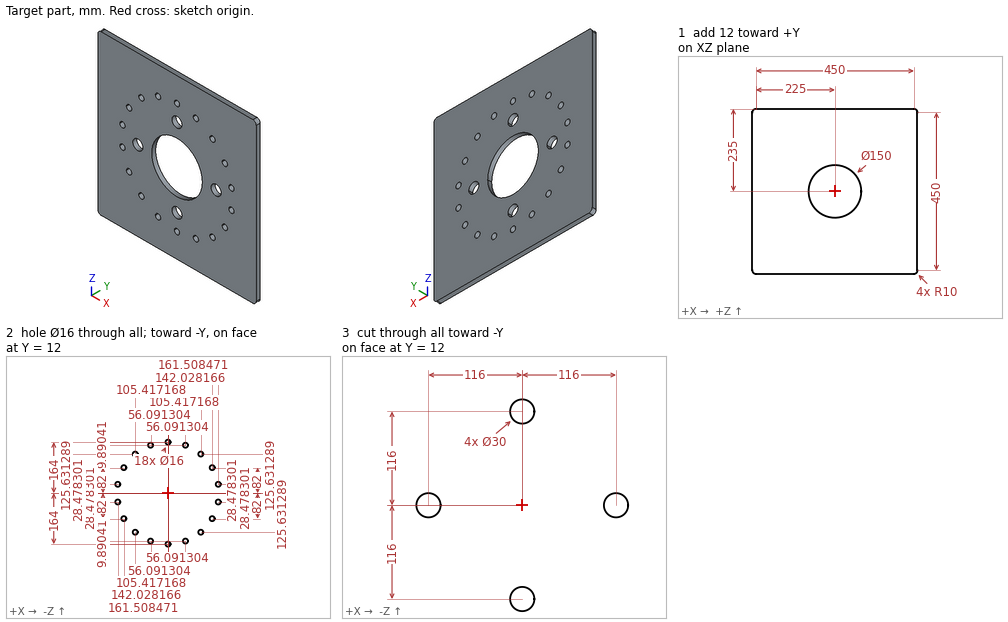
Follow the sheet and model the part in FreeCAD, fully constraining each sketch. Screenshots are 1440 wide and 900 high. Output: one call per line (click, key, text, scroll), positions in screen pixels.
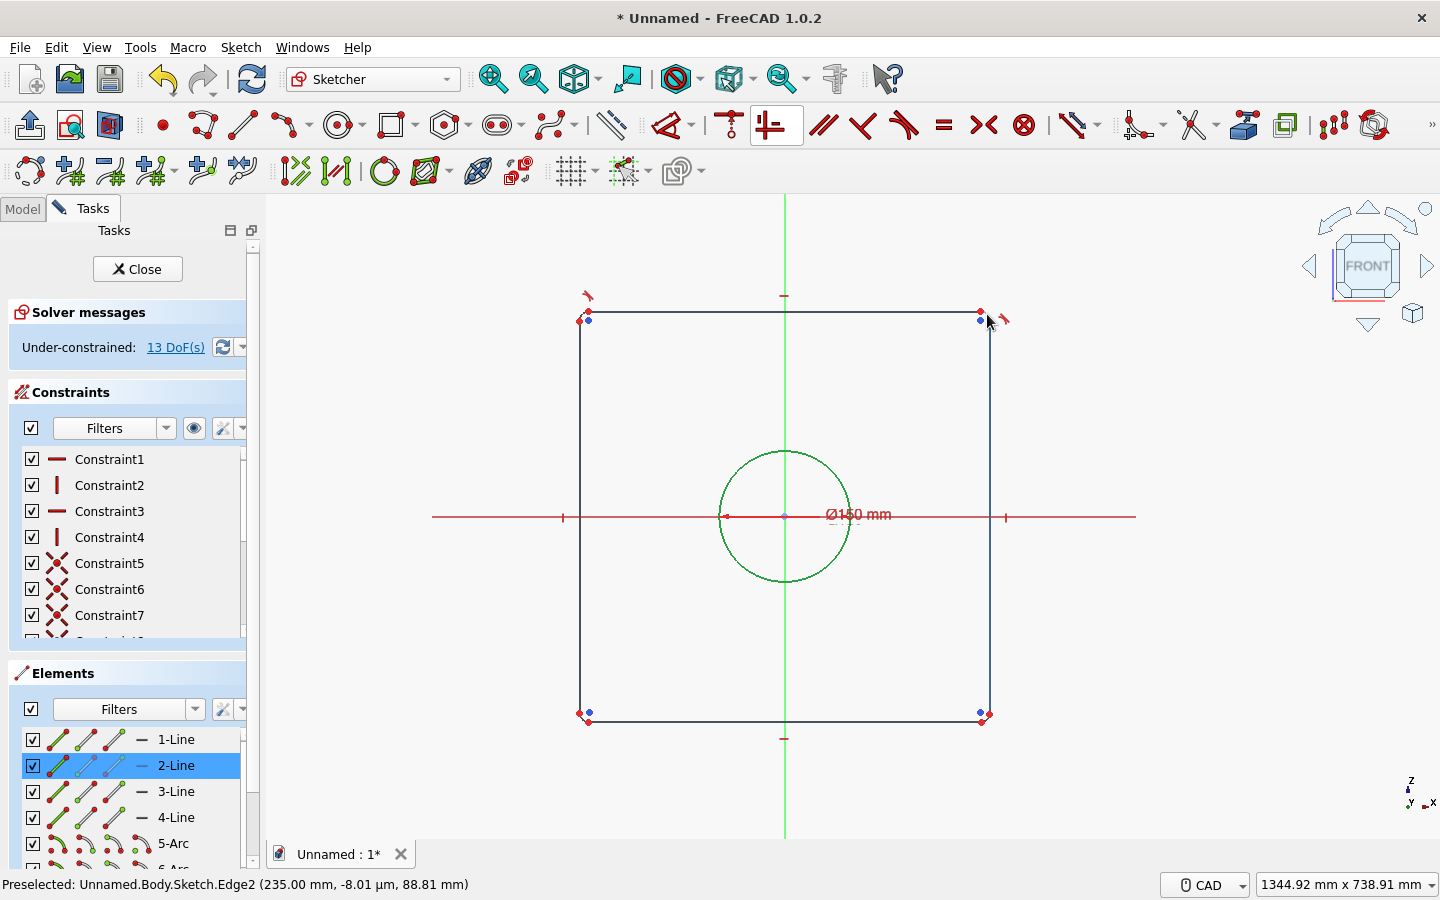
scroll(987, 720, up, 4)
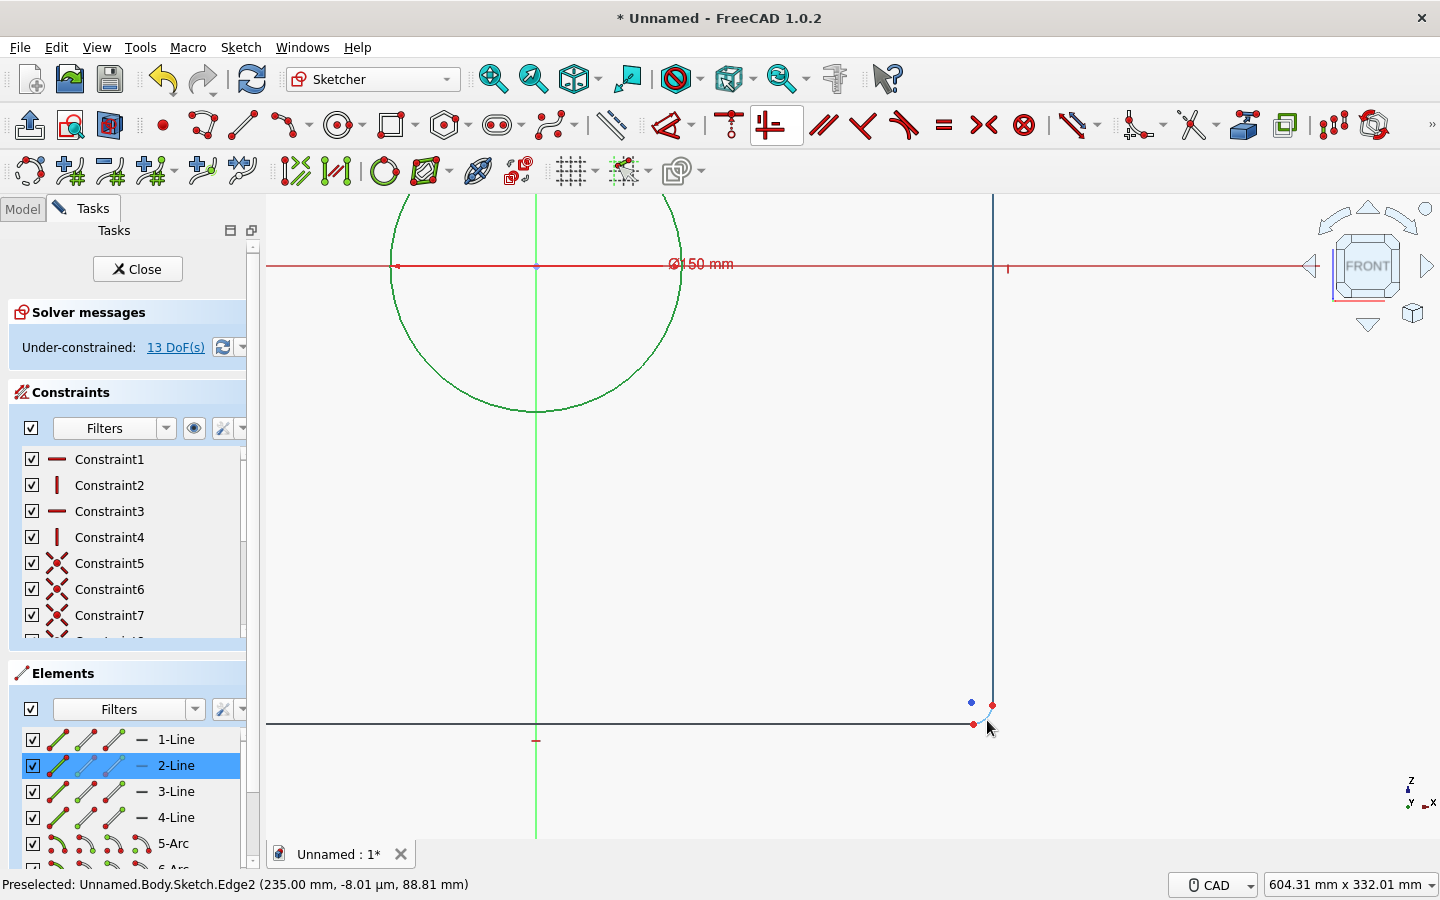
click(986, 718)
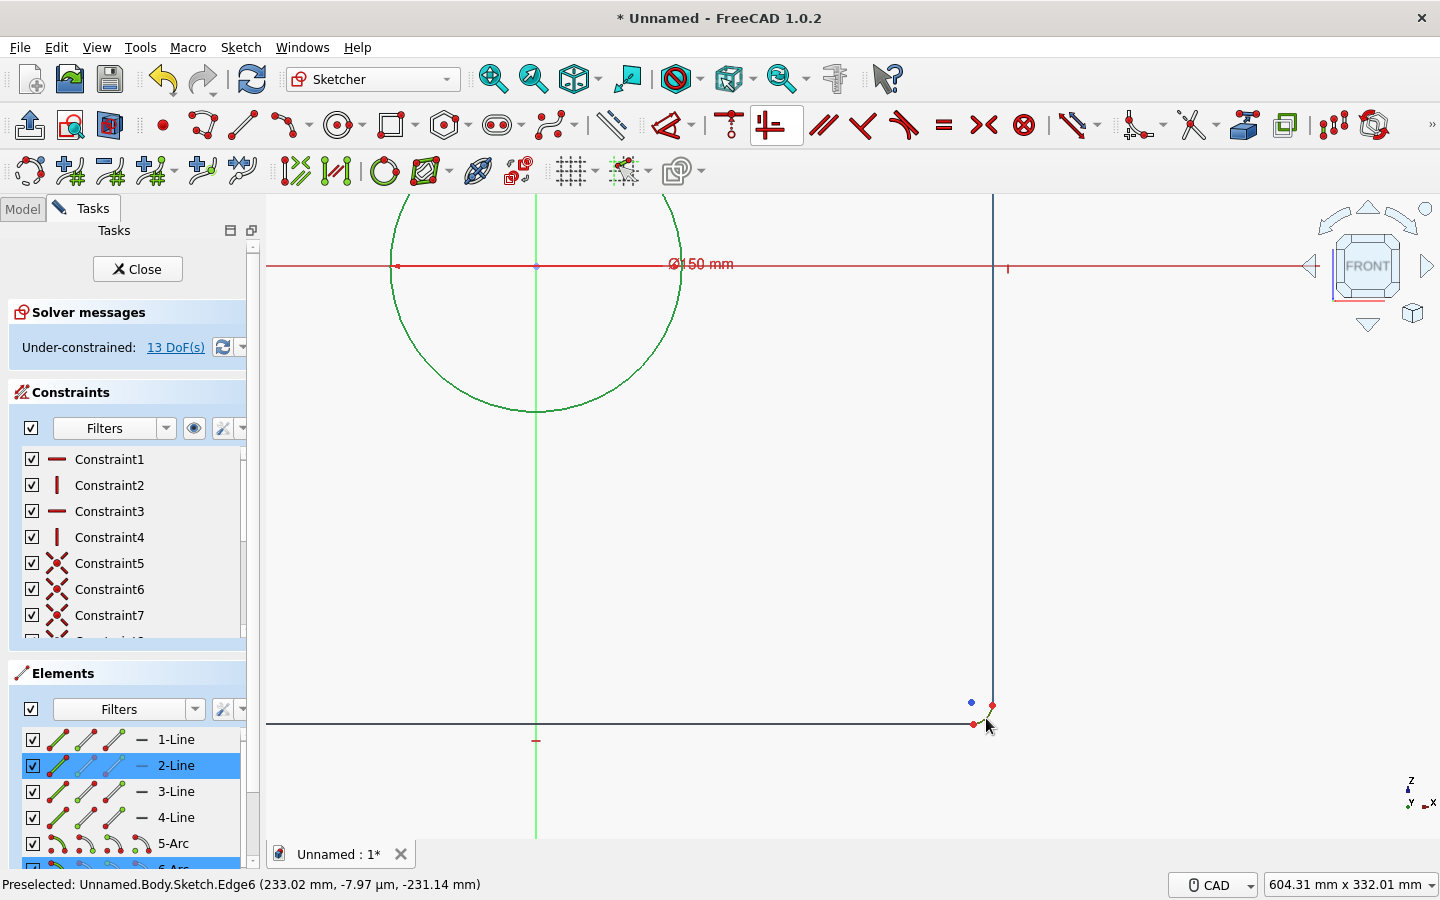
click(904, 126)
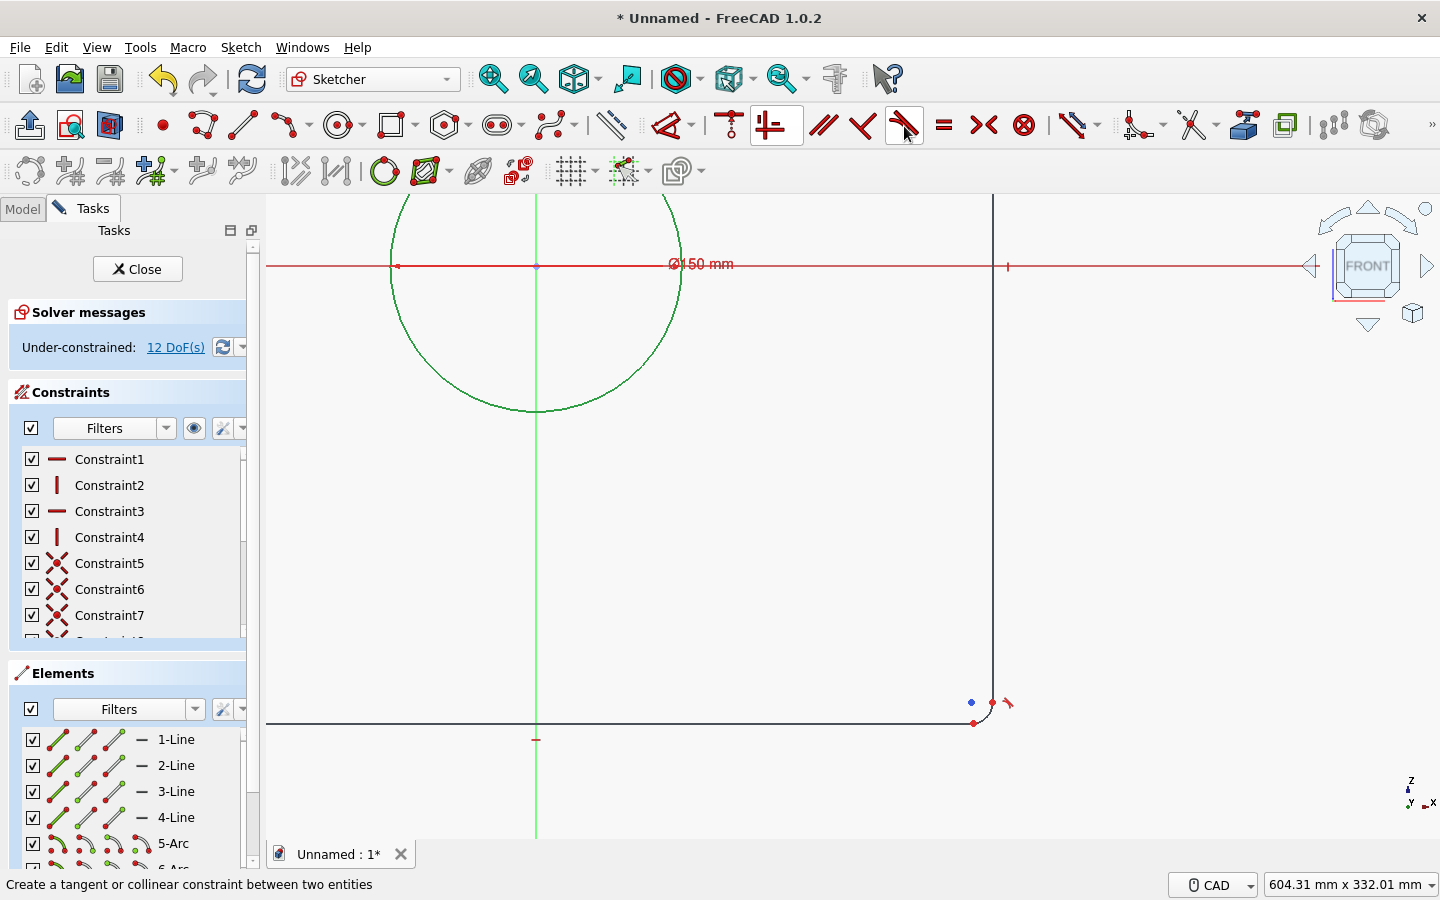
click(711, 724)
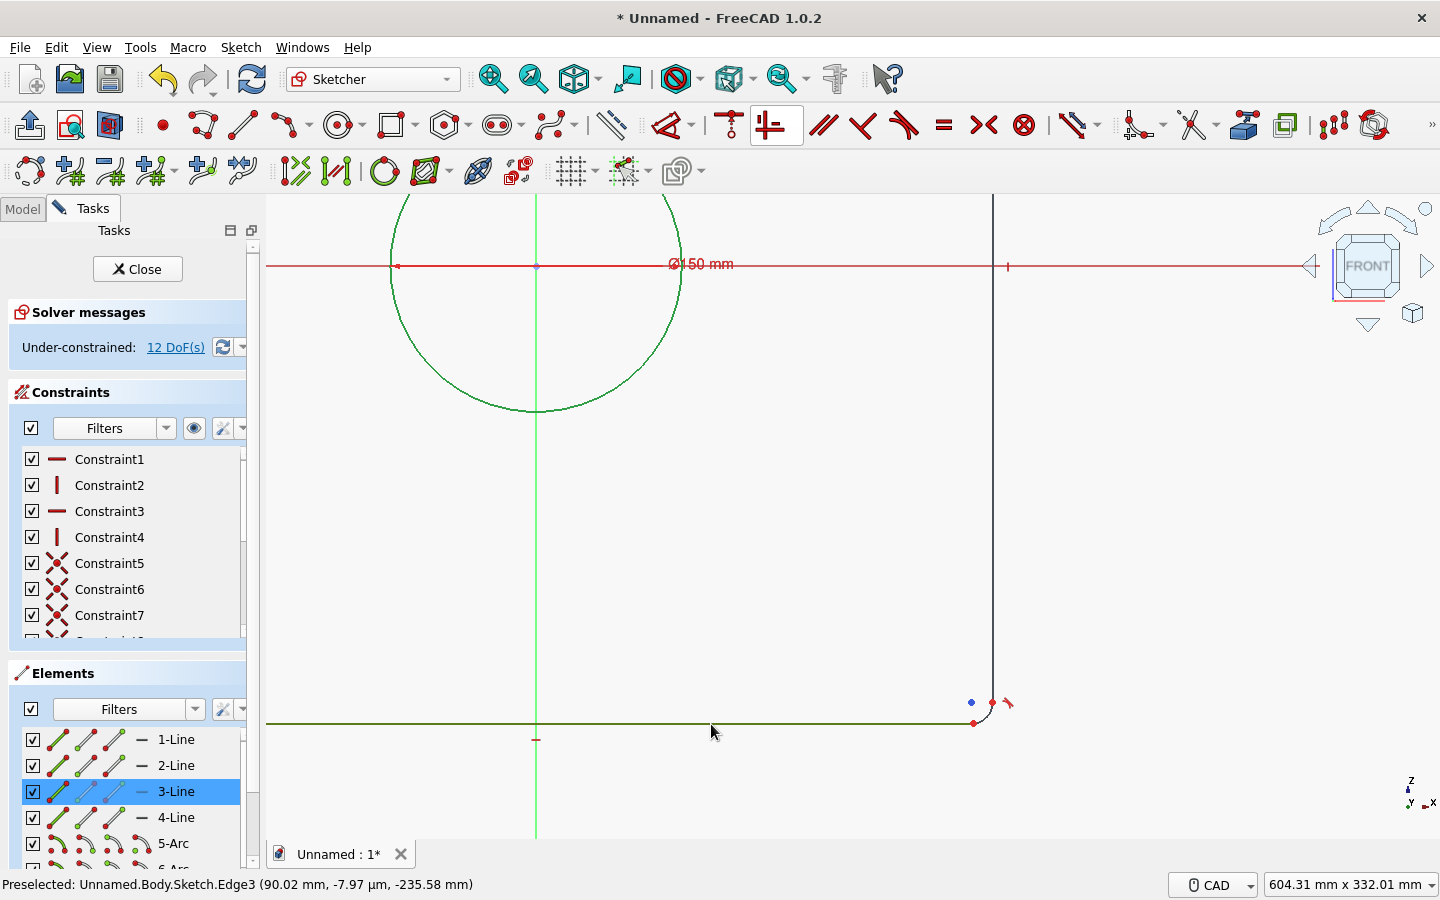
scroll(982, 721, up, 2)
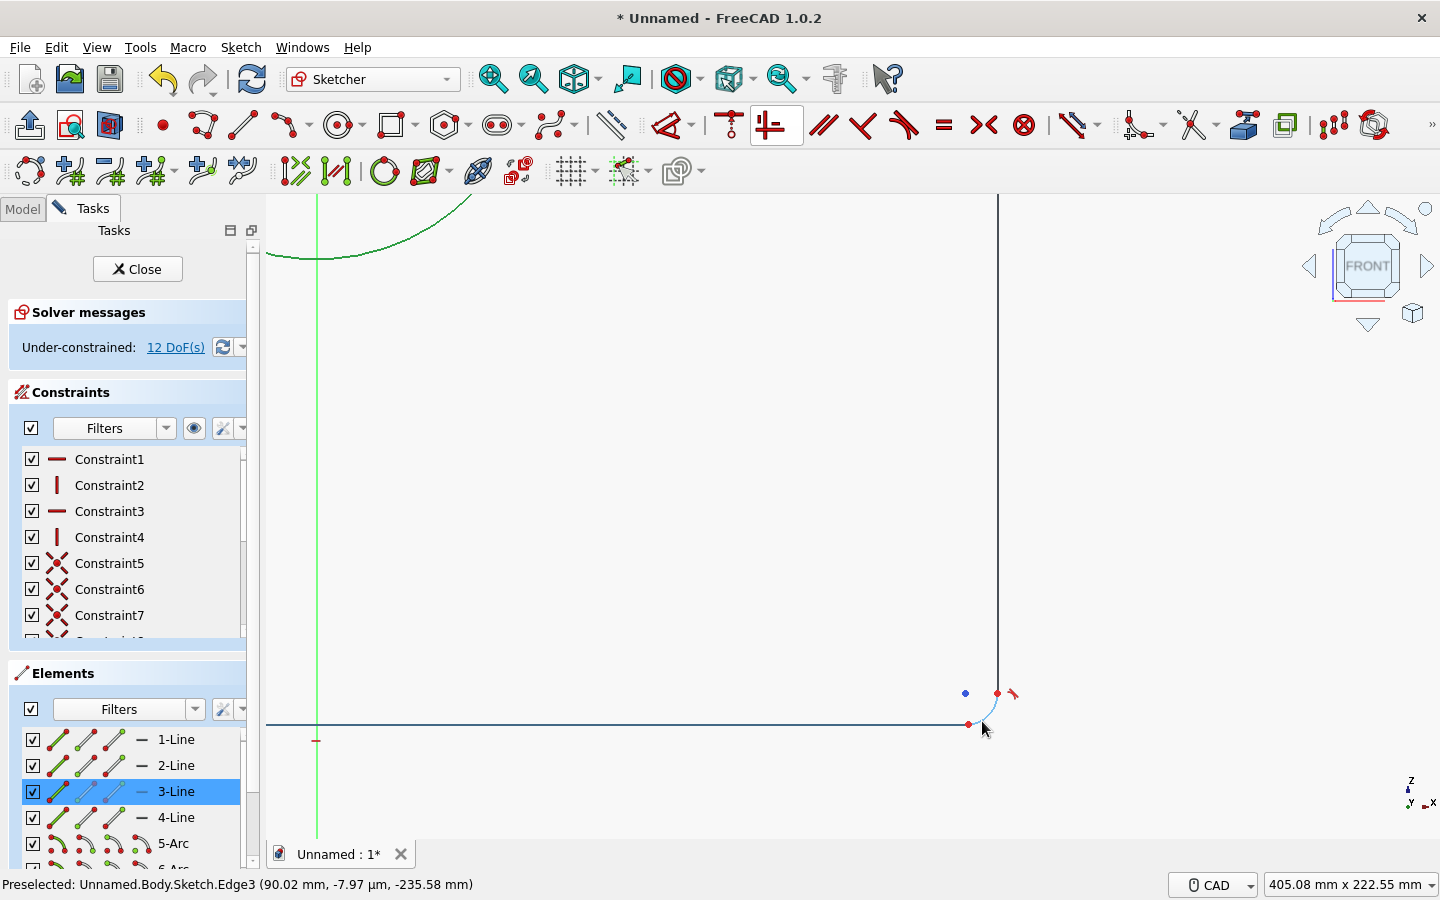
click(982, 720)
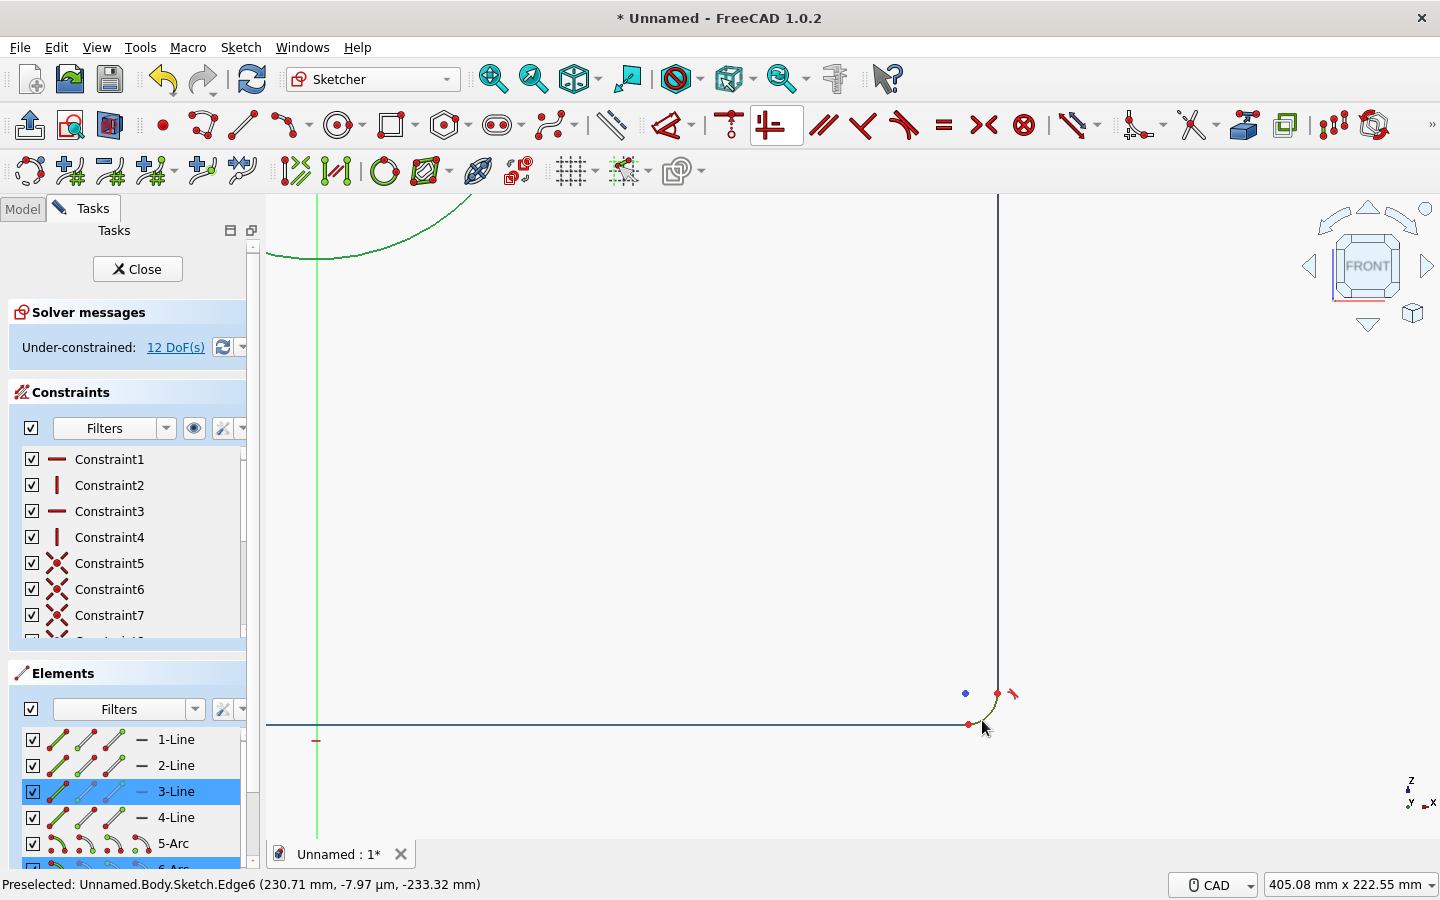
click(904, 126)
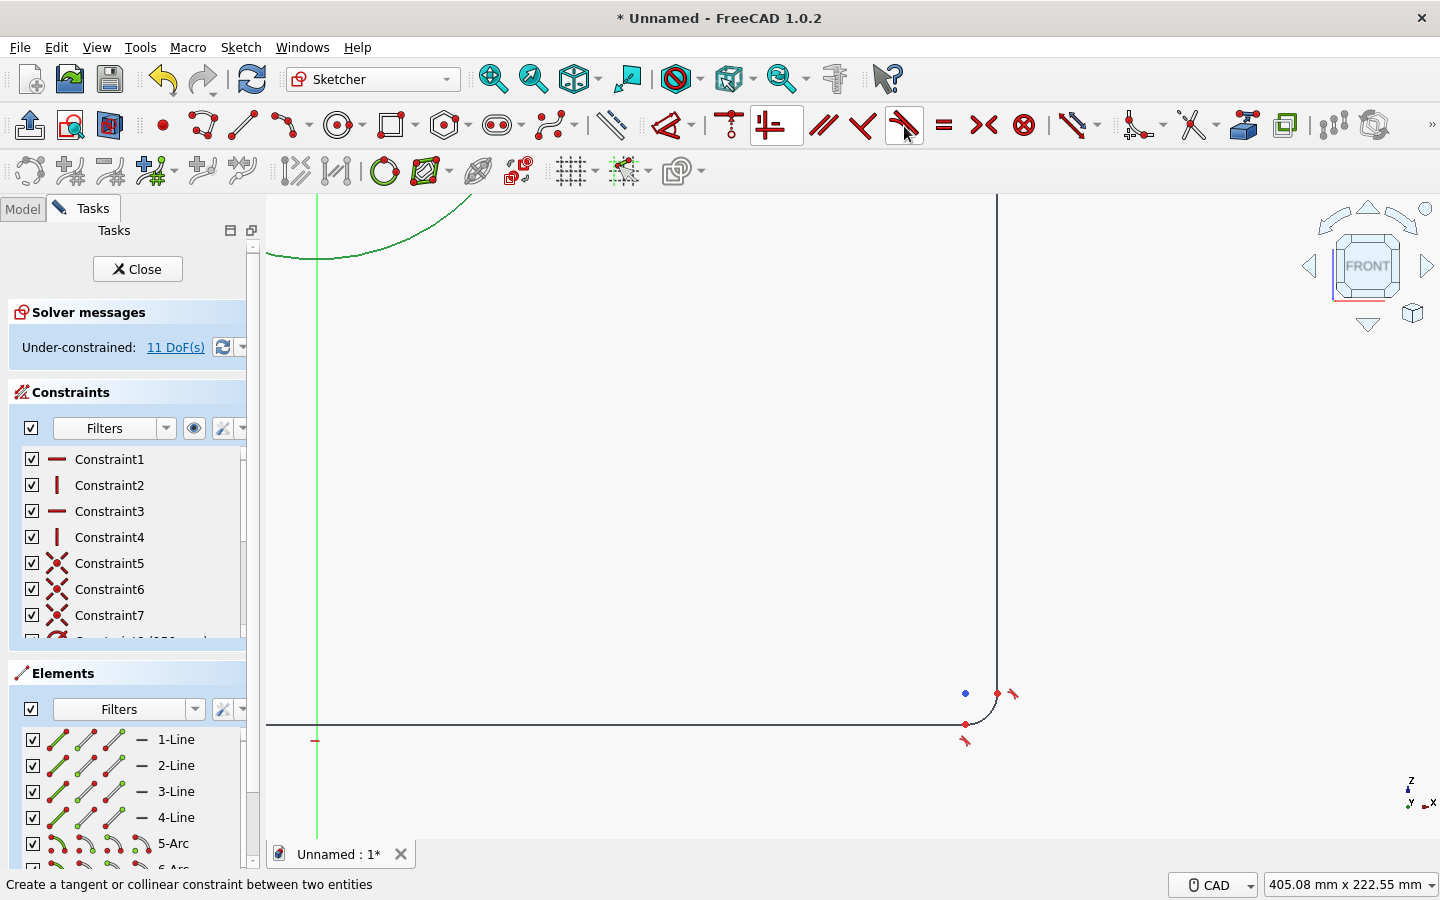
click(575, 725)